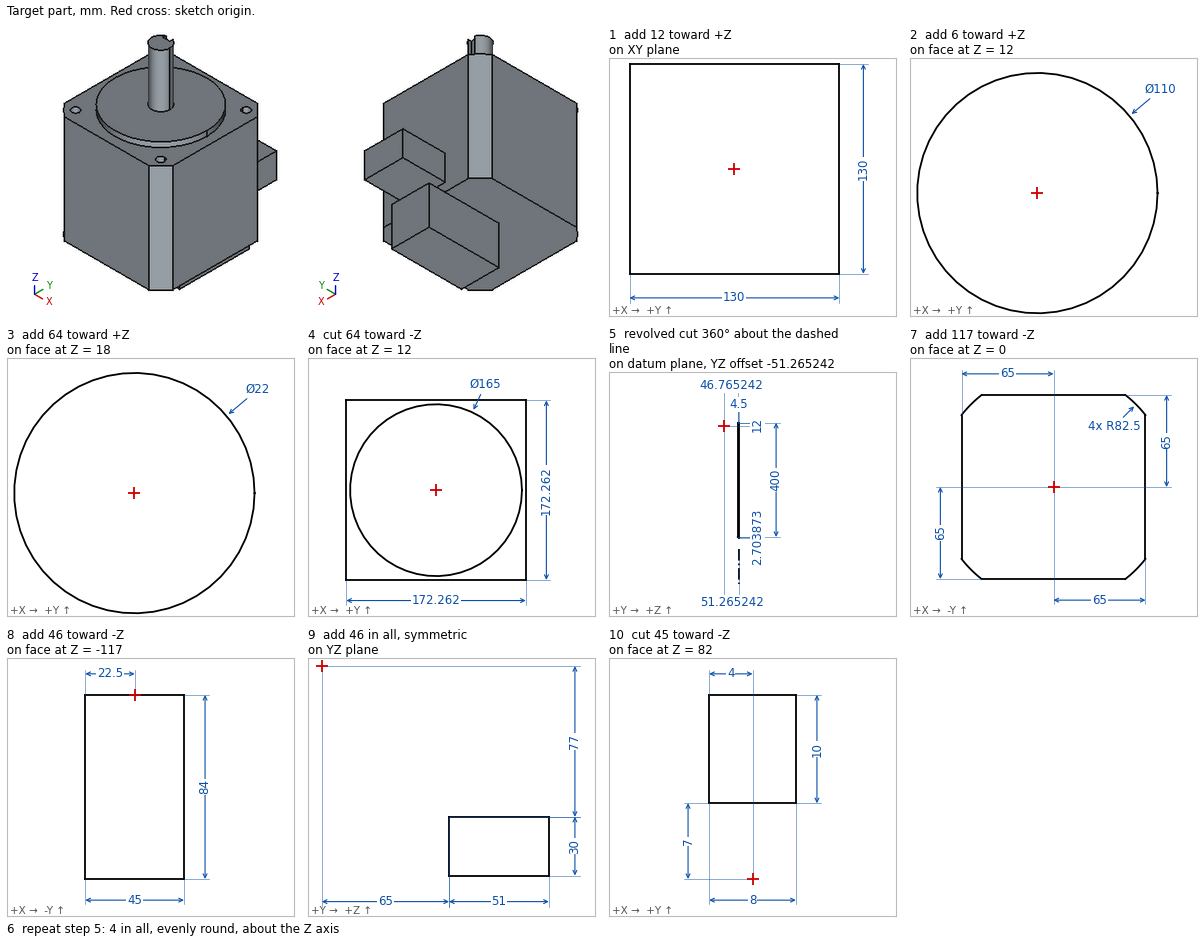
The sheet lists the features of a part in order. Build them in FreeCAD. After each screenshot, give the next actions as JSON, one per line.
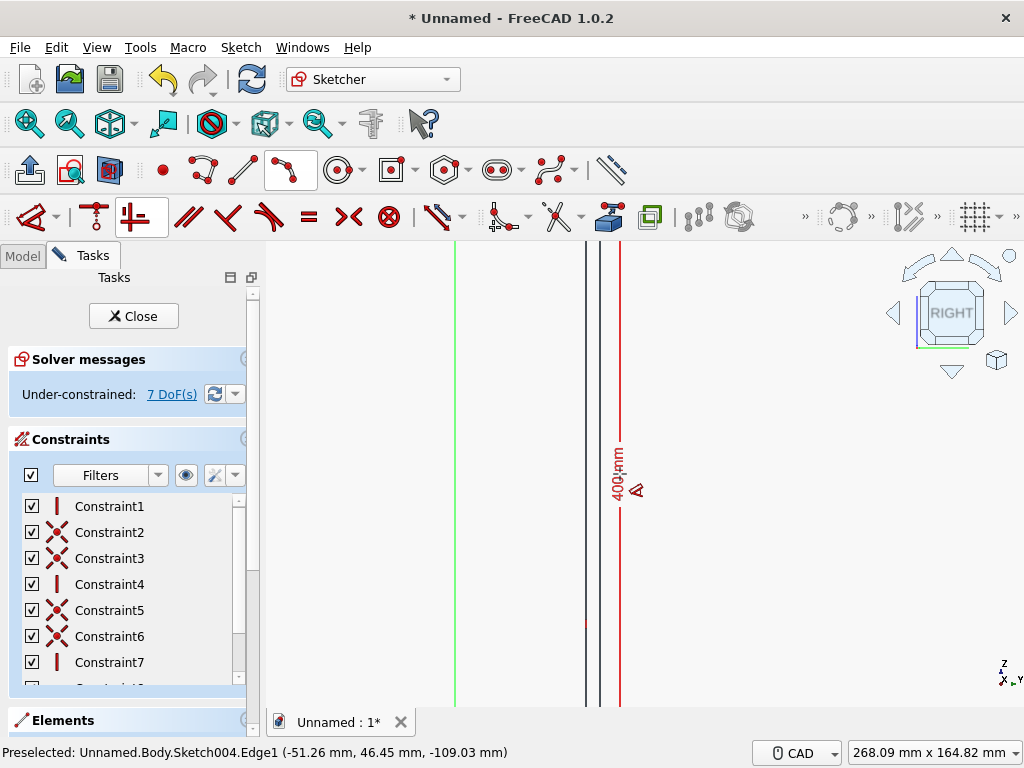
{"action": "scroll", "coordinate": [586, 399], "scroll_direction": "down", "scroll_amount": 9}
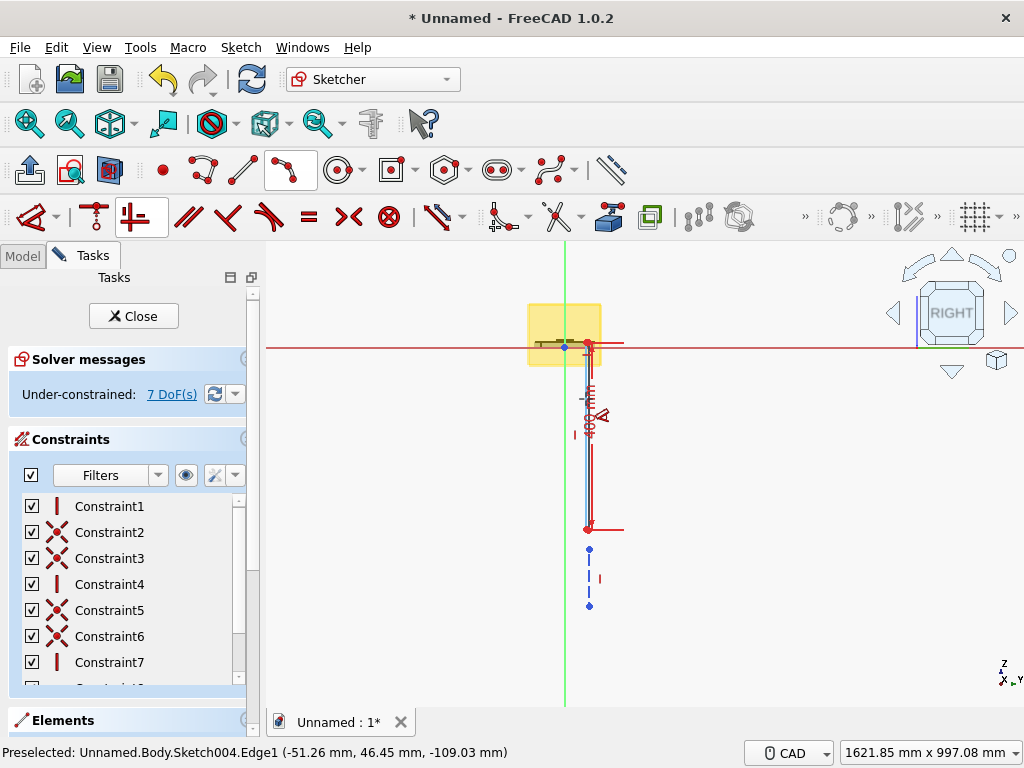
{"action": "scroll", "coordinate": [588, 343], "scroll_direction": "up", "scroll_amount": 15}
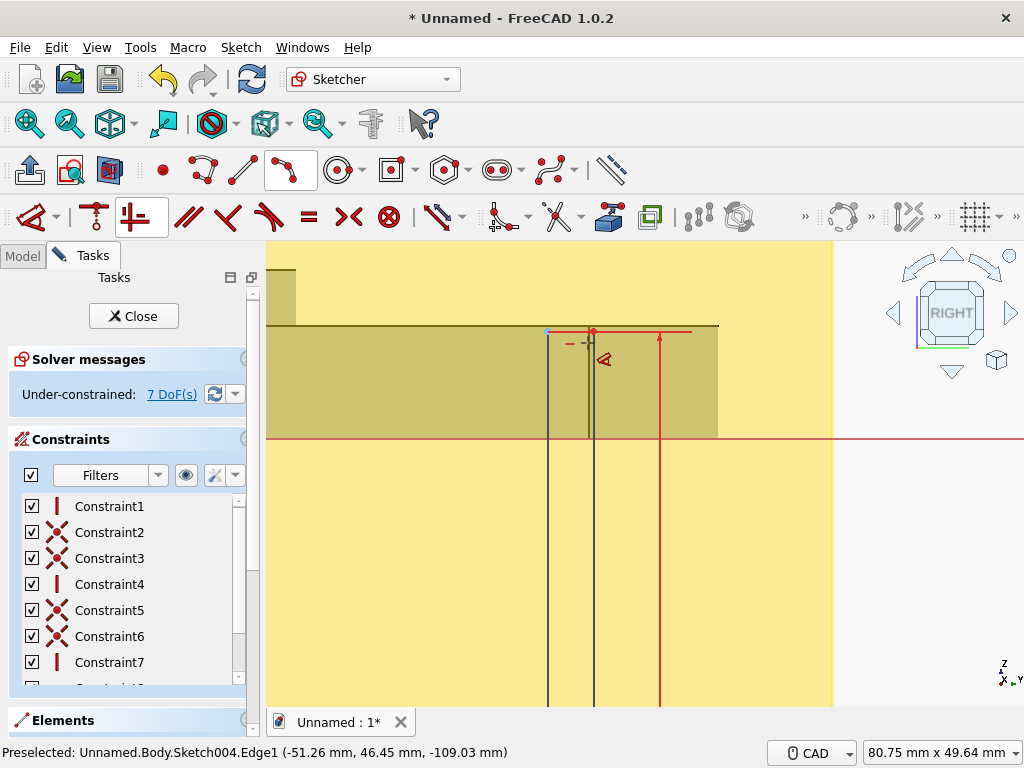
{"action": "left_click", "coordinate": [571, 332]}
{"action": "left_click", "coordinate": [571, 298]}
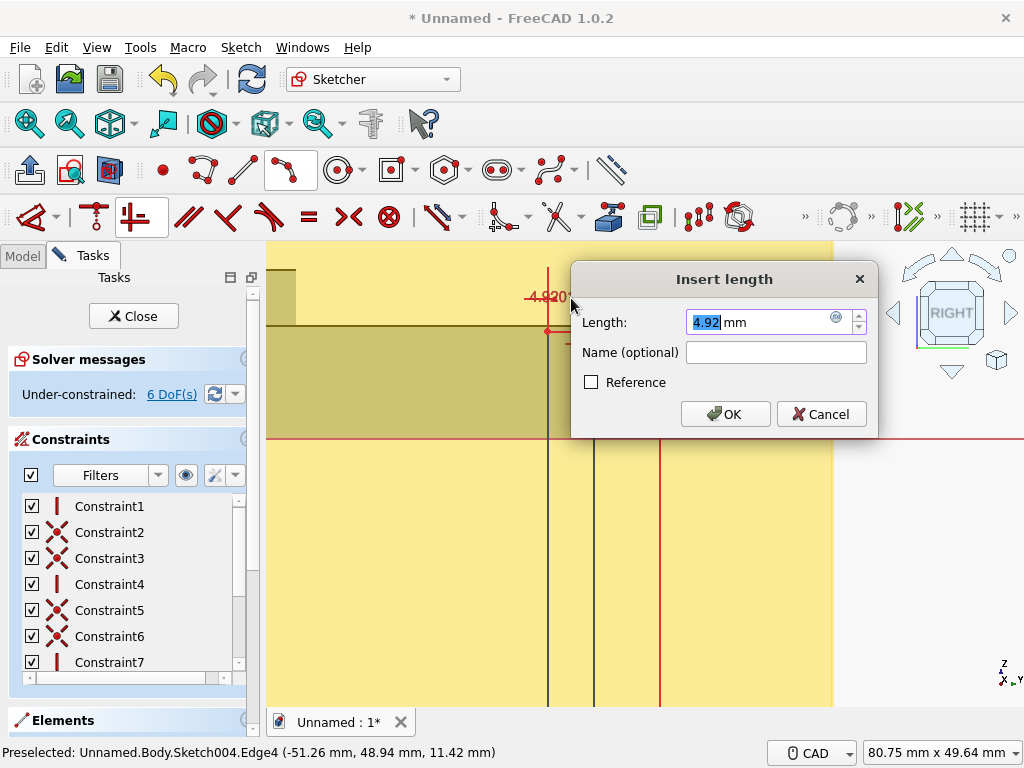
{"action": "type", "text": "4.5"}
{"action": "key", "text": "Return"}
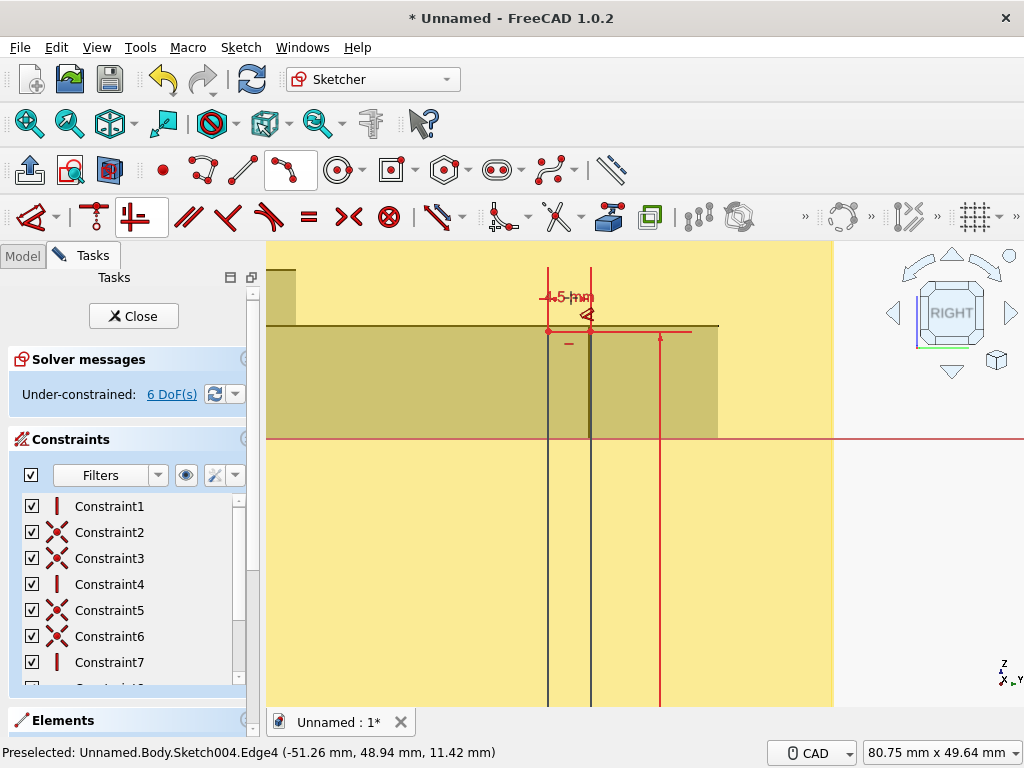
{"action": "left_click", "coordinate": [548, 332]}
{"action": "left_click", "coordinate": [606, 386]}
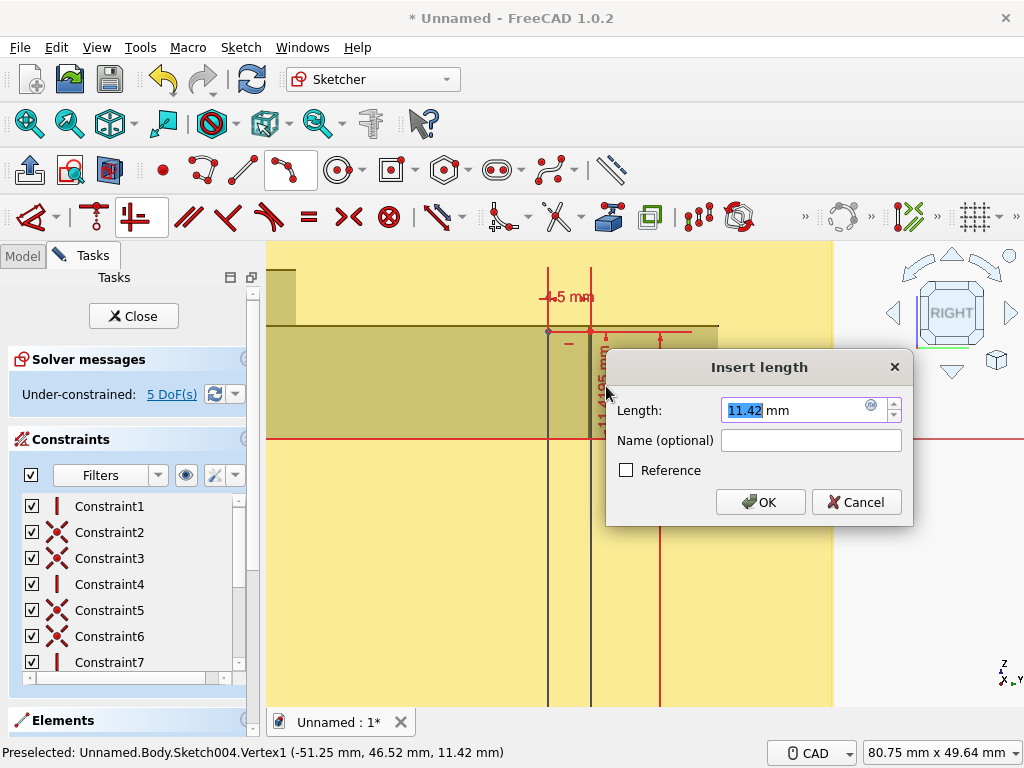
{"action": "type", "text": "12"}
{"action": "key", "text": "Return"}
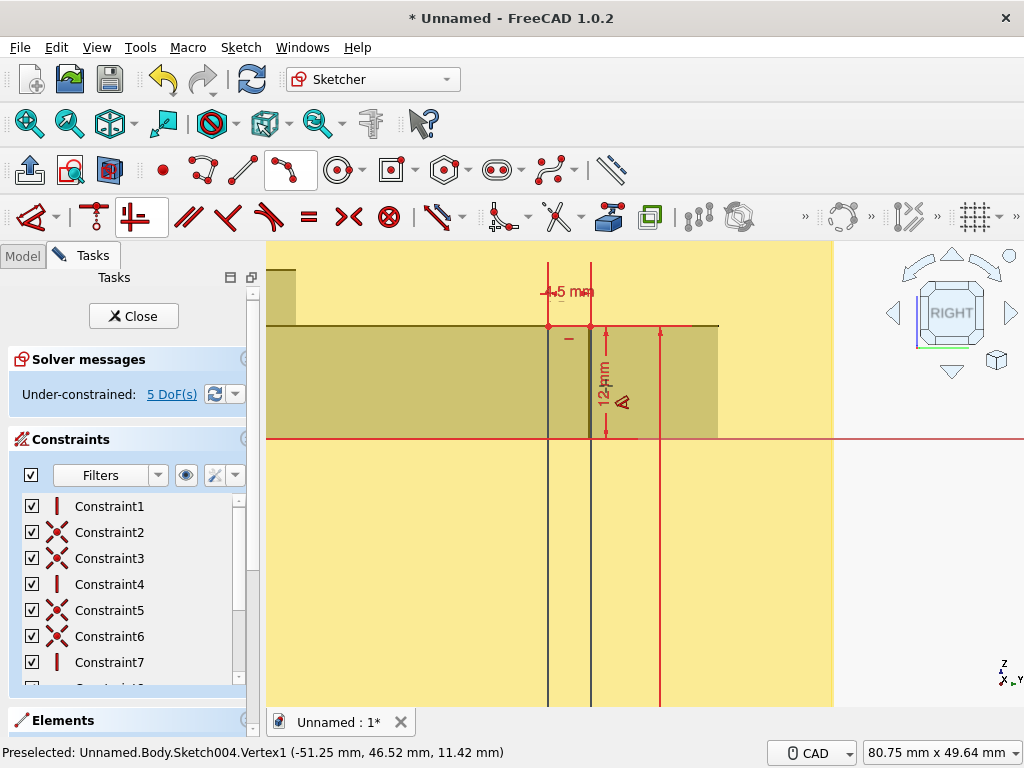
{"action": "scroll", "coordinate": [588, 343], "scroll_direction": "down", "scroll_amount": 15}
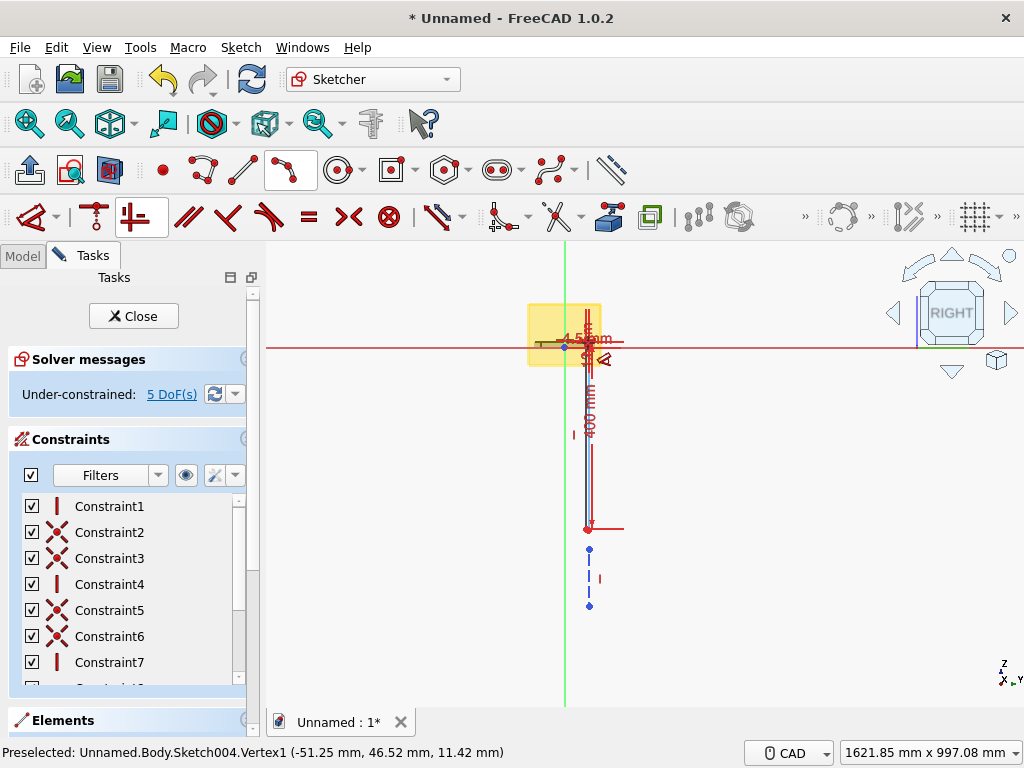
{"action": "scroll", "coordinate": [587, 530], "scroll_direction": "up", "scroll_amount": 18}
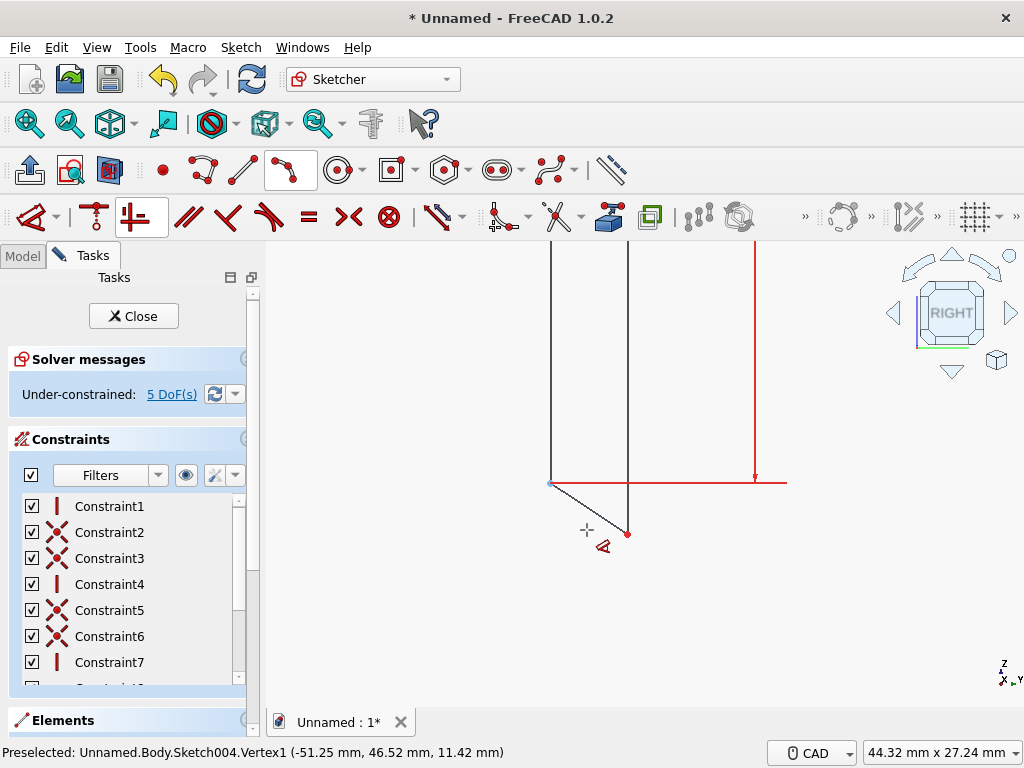
{"action": "left_click", "coordinate": [574, 499]}
{"action": "left_click", "coordinate": [662, 509]}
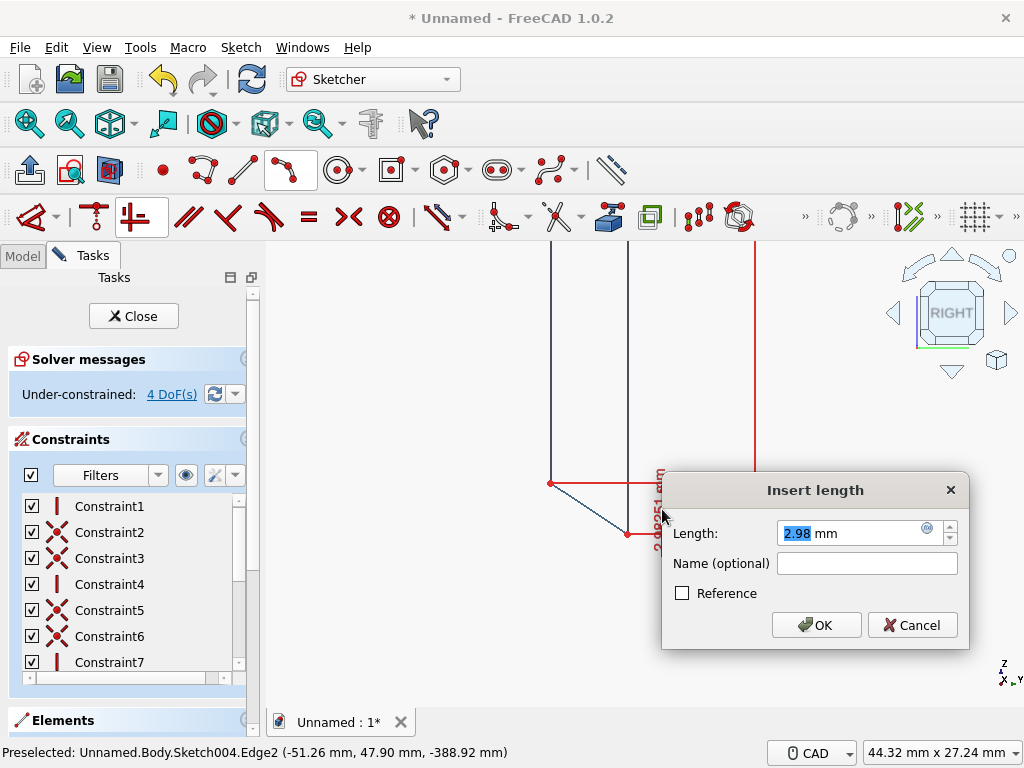
{"action": "type", "text": "2.703873"}
{"action": "key", "text": "Return"}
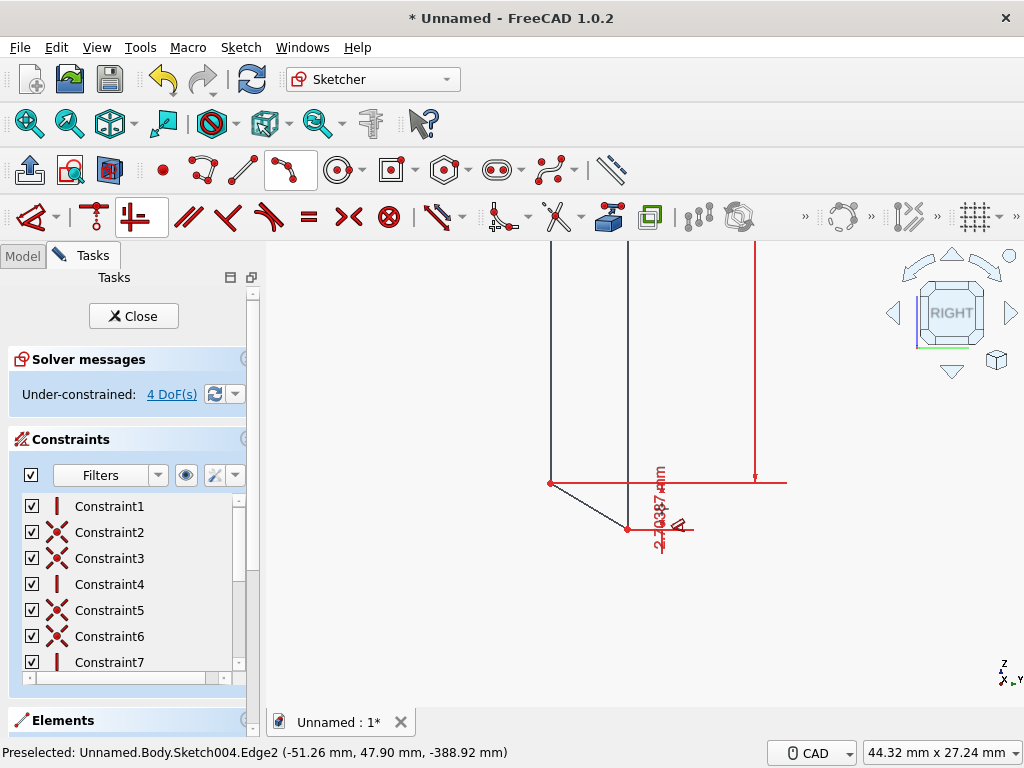
{"action": "scroll", "coordinate": [590, 543], "scroll_direction": "down", "scroll_amount": 17}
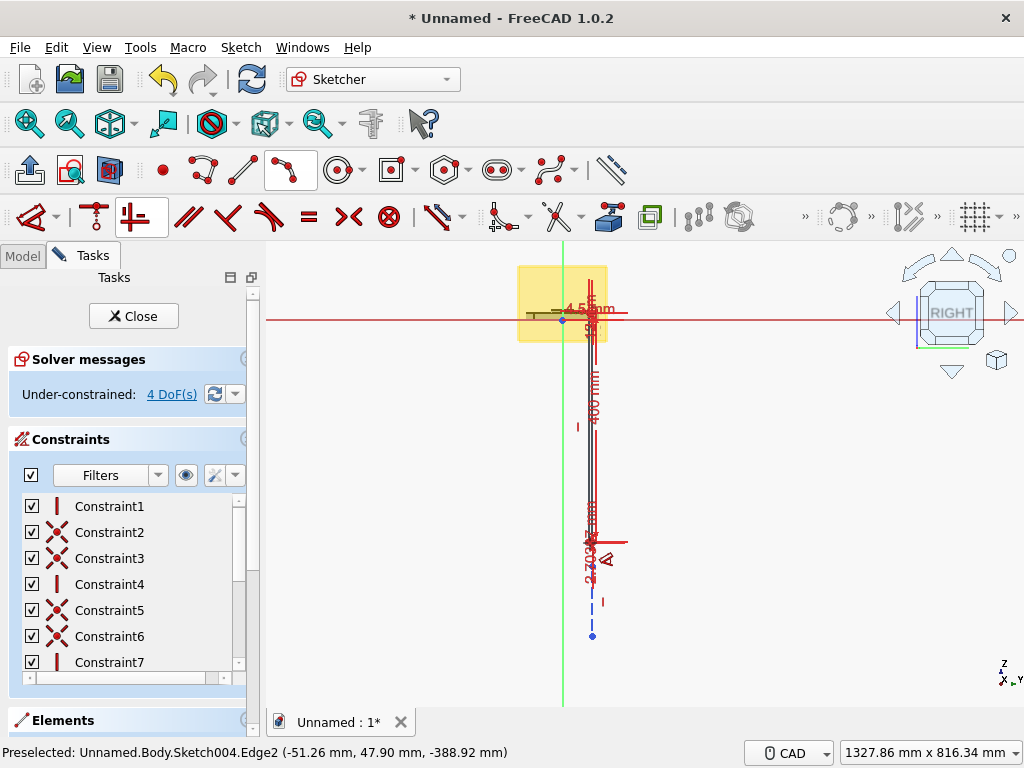
{"action": "scroll", "coordinate": [589, 313], "scroll_direction": "up", "scroll_amount": 8}